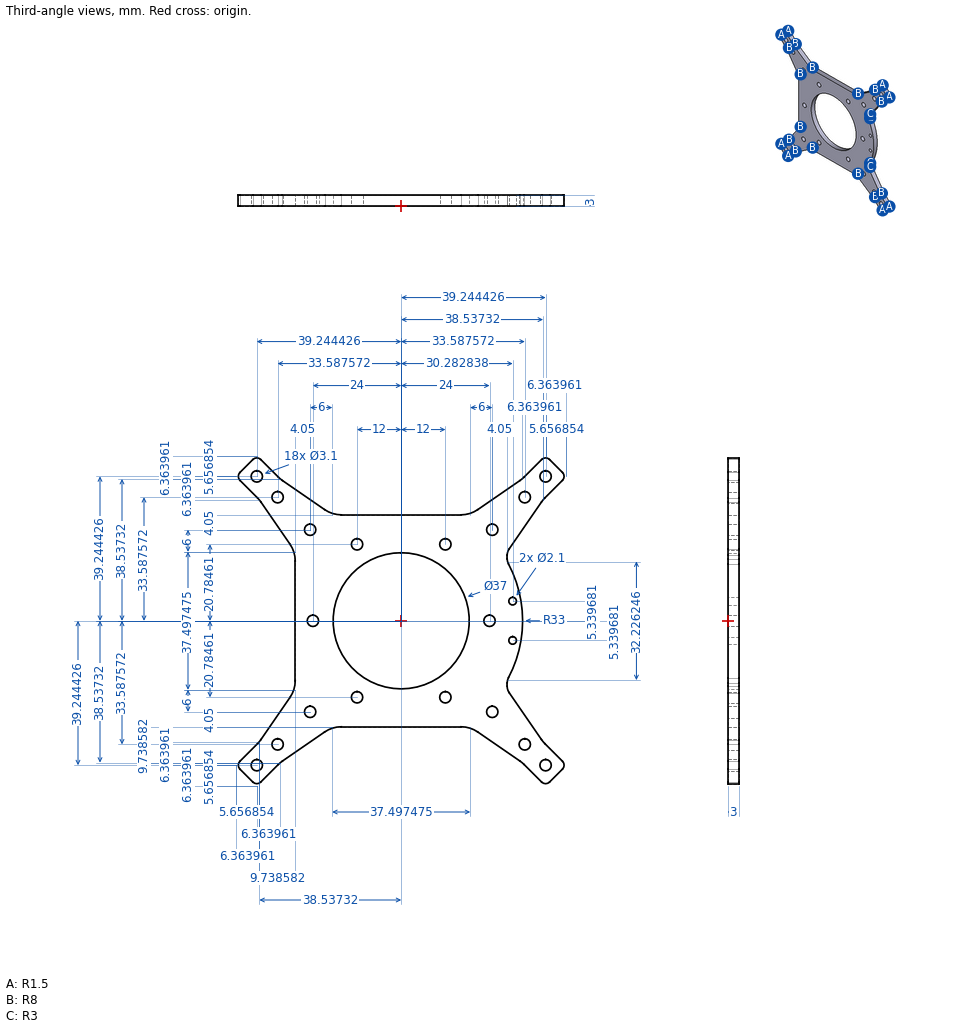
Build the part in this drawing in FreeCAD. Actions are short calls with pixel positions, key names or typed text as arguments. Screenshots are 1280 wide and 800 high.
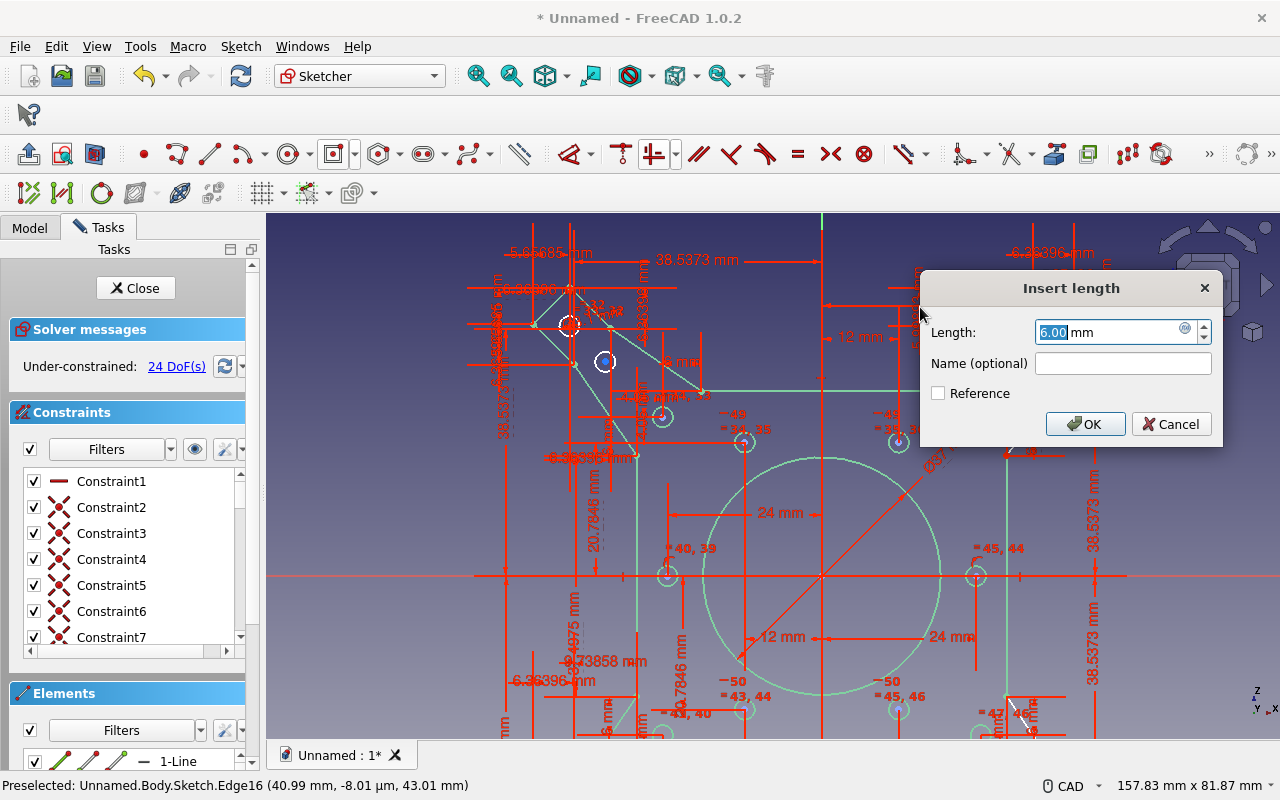
text(5.656854)
key(Return)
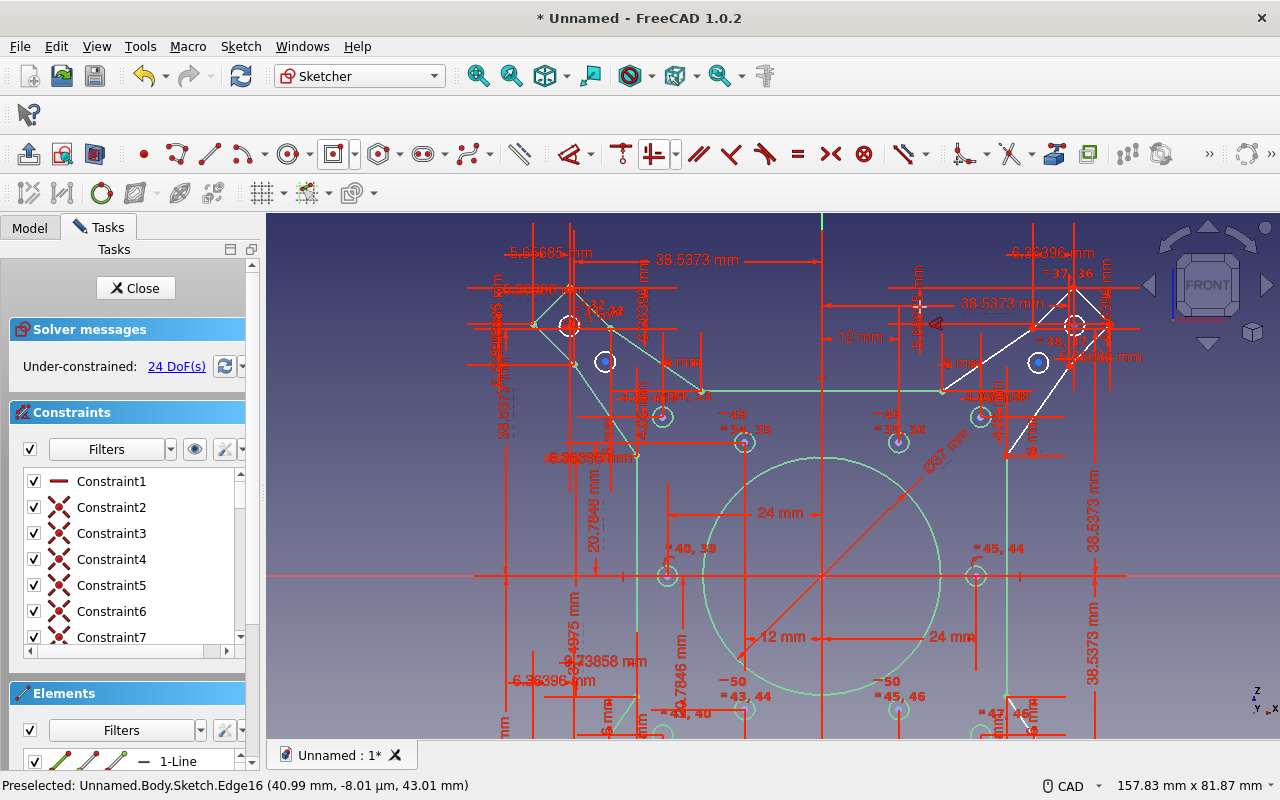
click(1098, 337)
click(1090, 400)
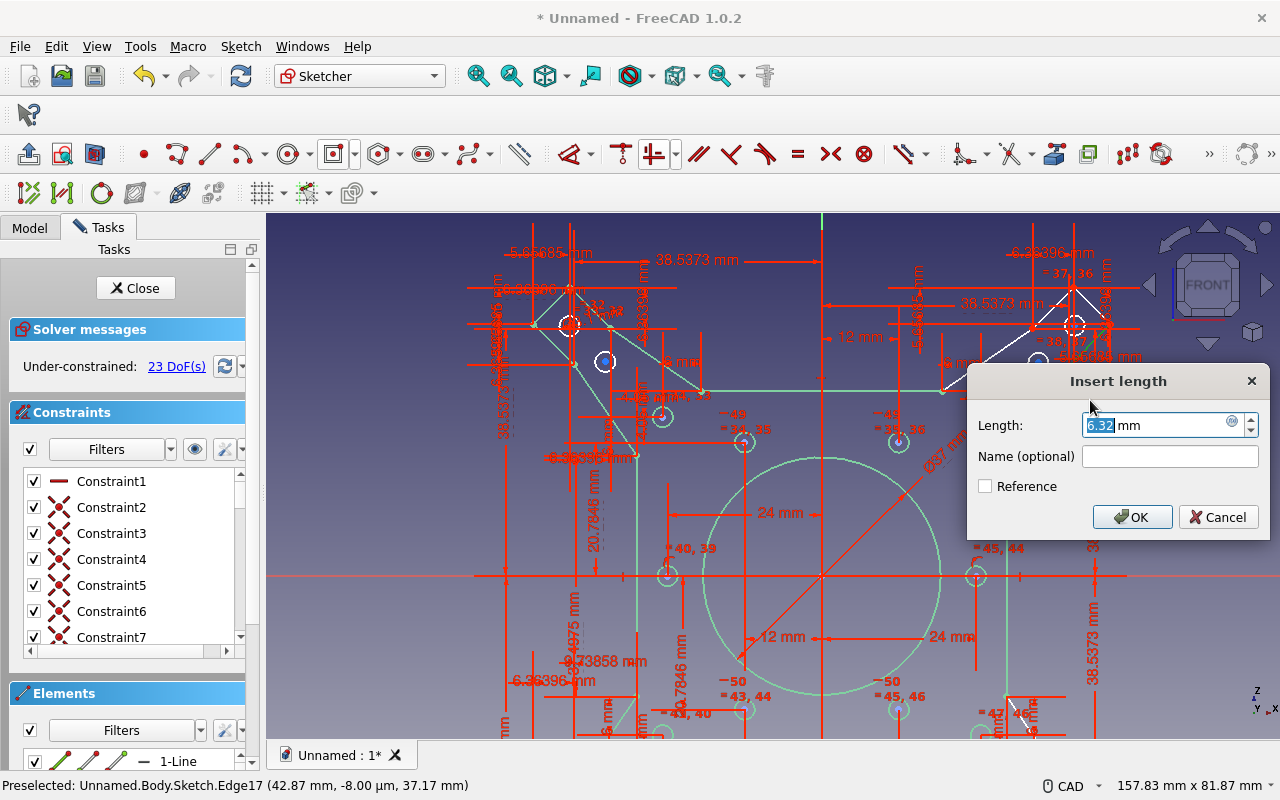
text(6.363961)
key(Return)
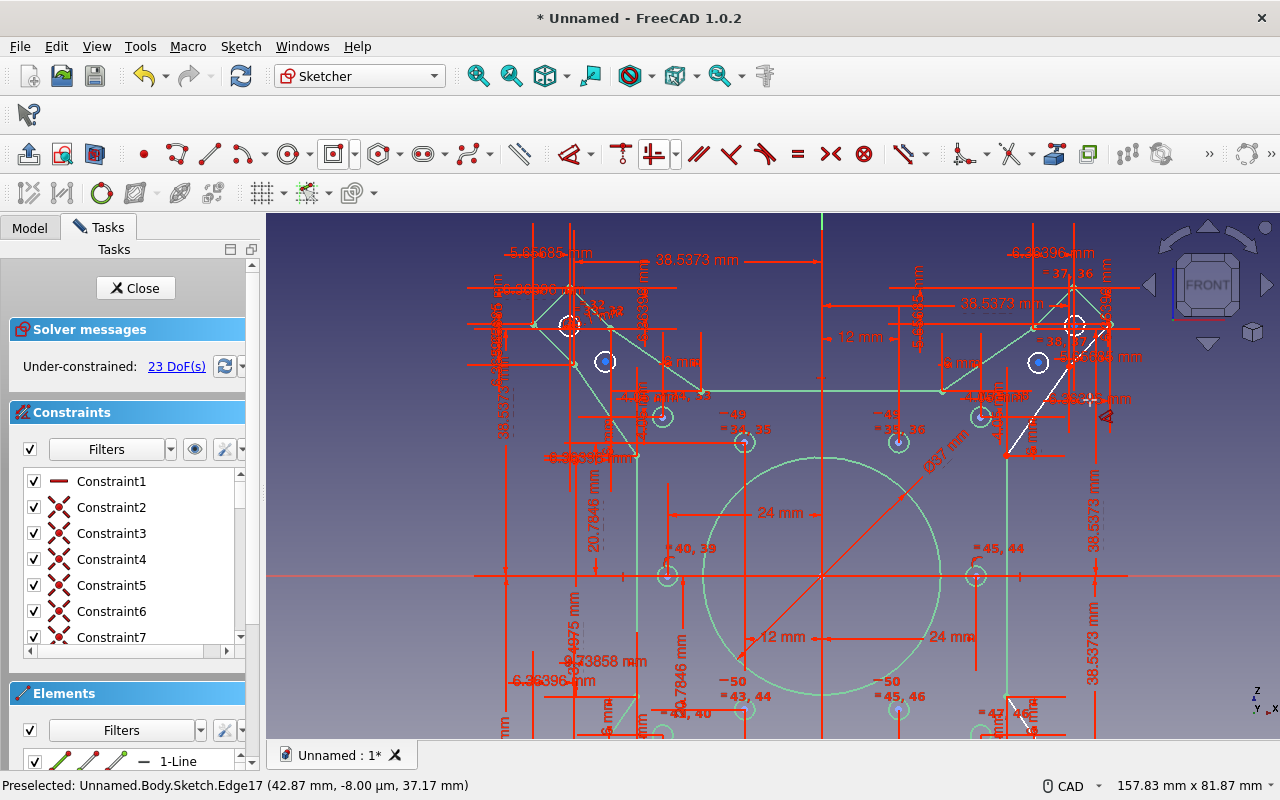
click(1098, 337)
click(987, 335)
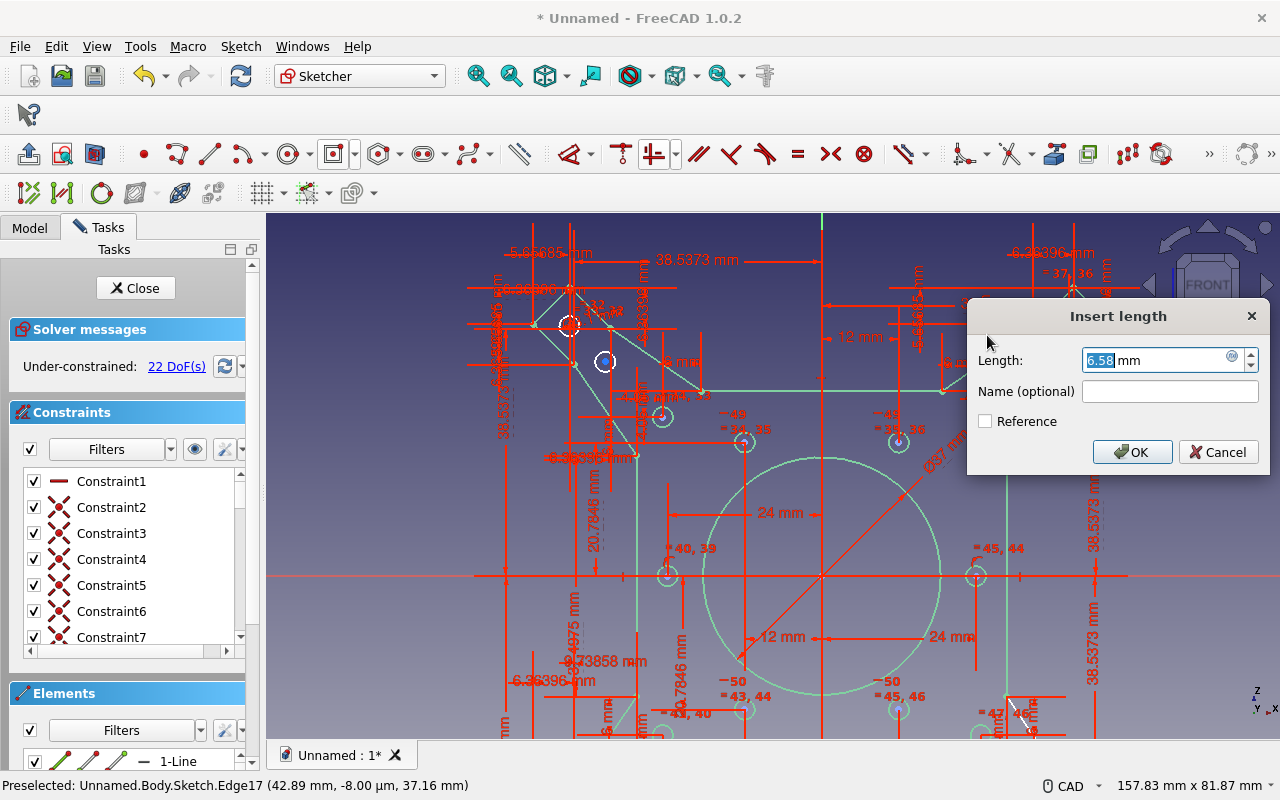
text(6.363961)
key(Return)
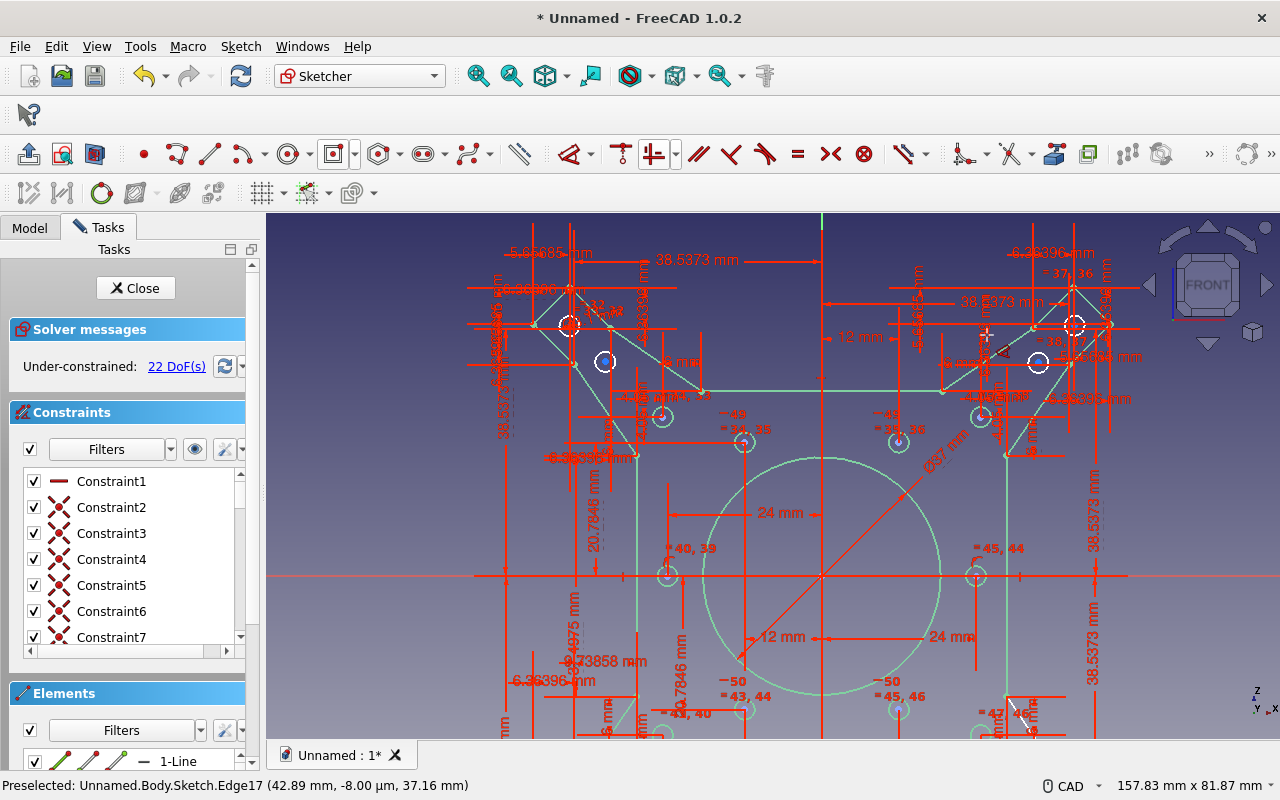
scroll(562, 354, down, 3)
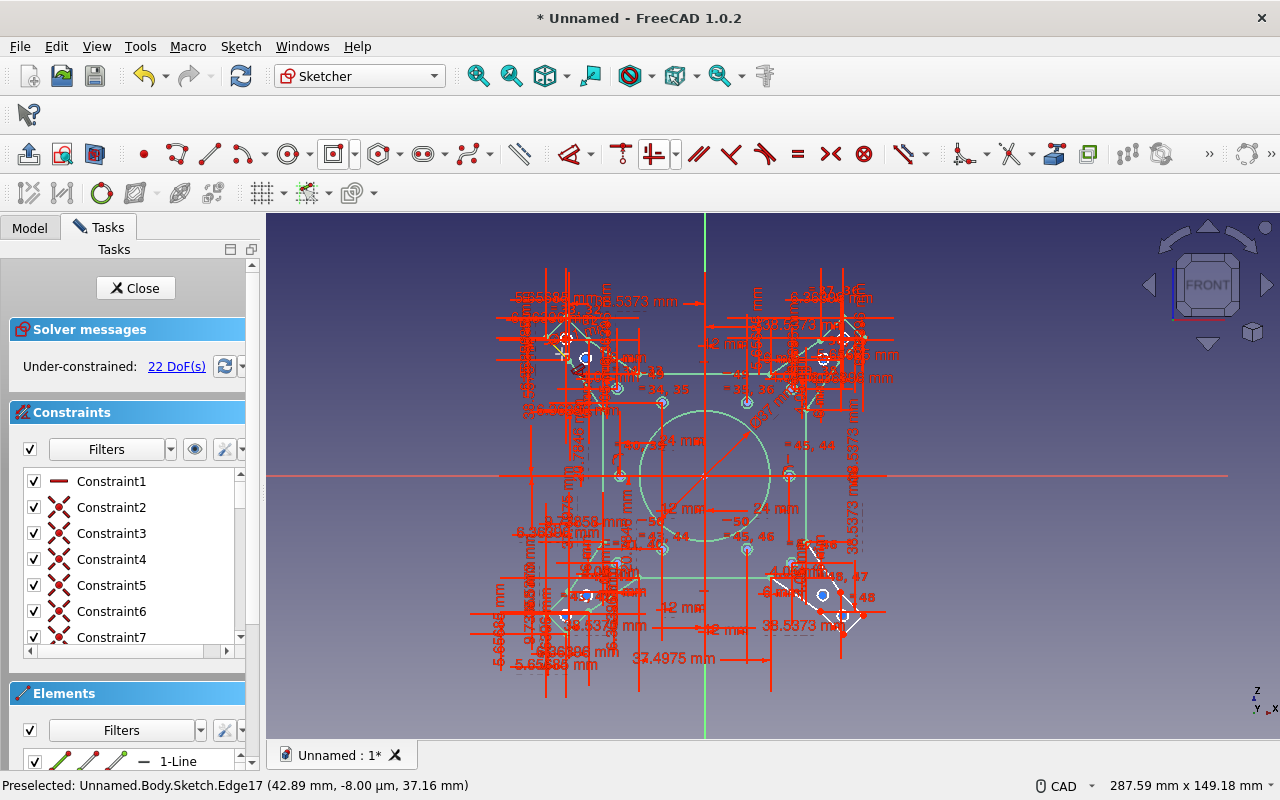
scroll(847, 600, up, 3)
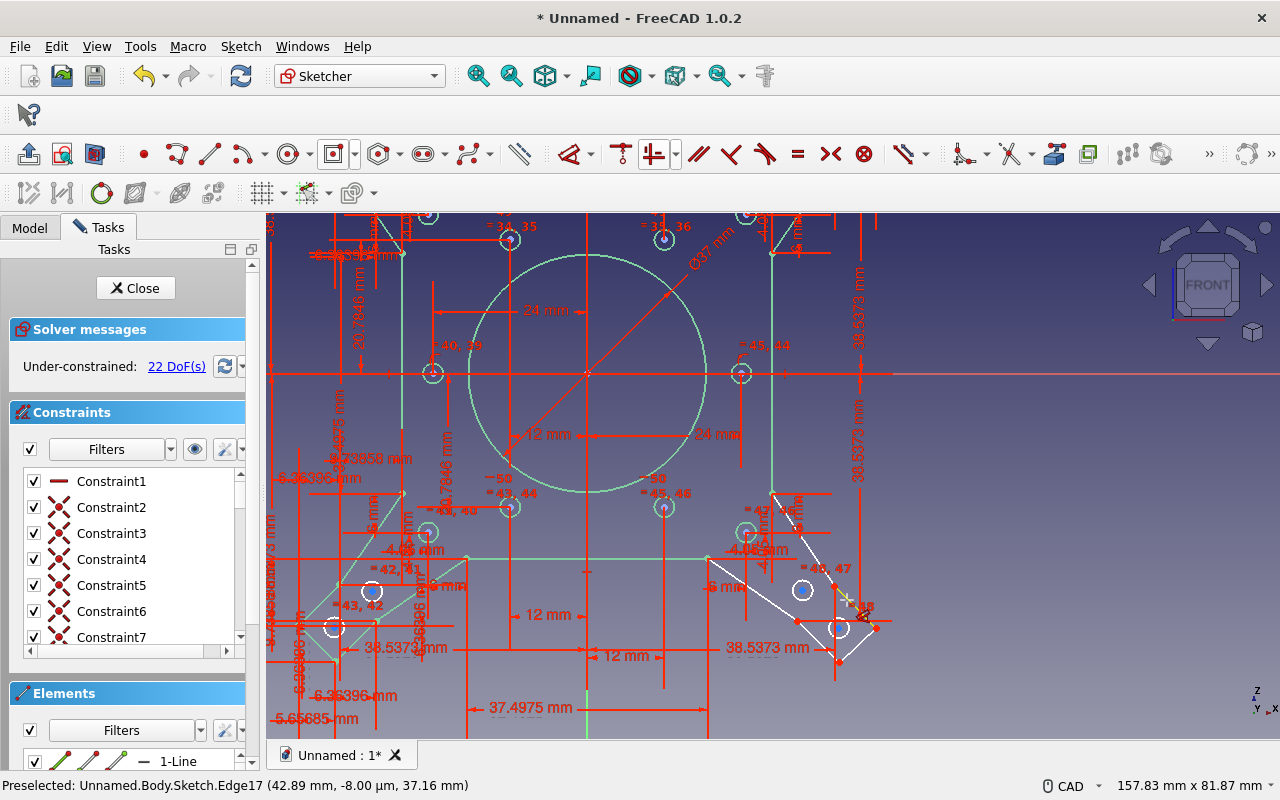
click(847, 599)
click(865, 662)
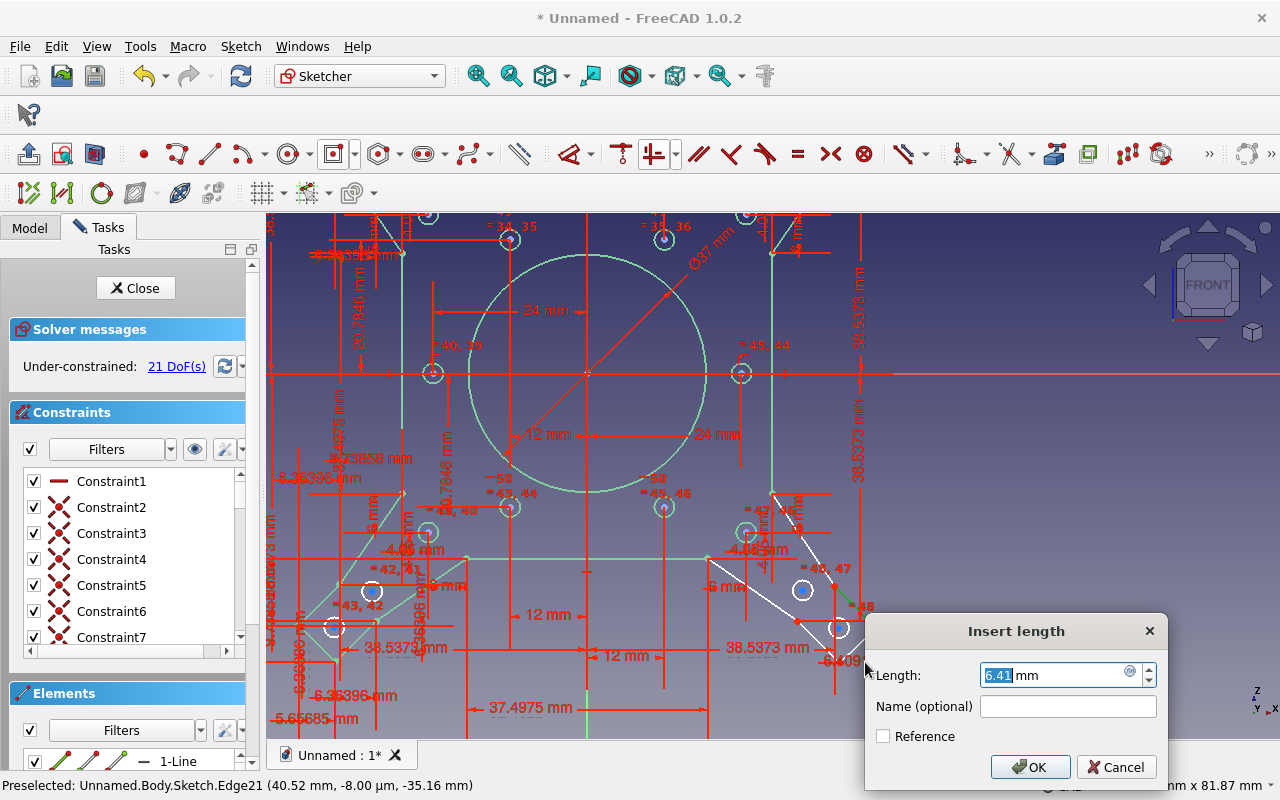
text(6.363961)
key(Return)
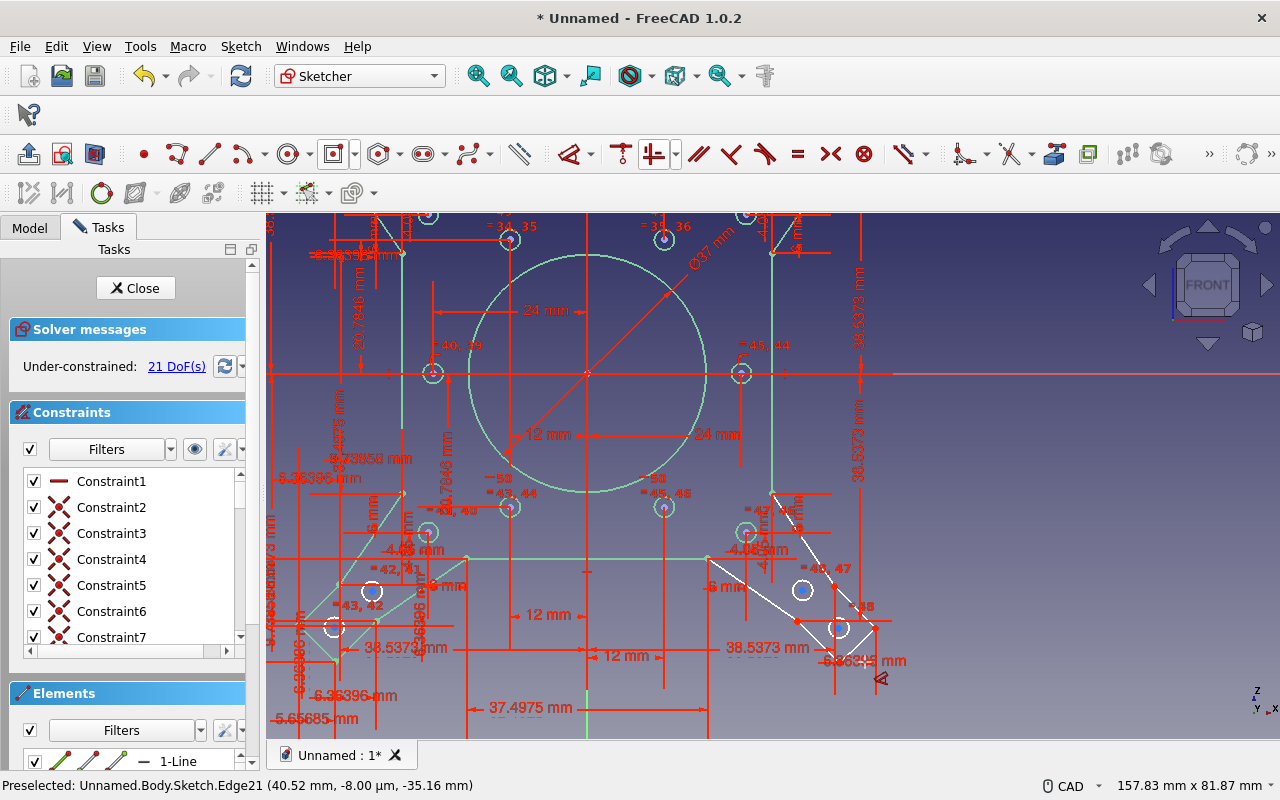
click(847, 599)
click(910, 607)